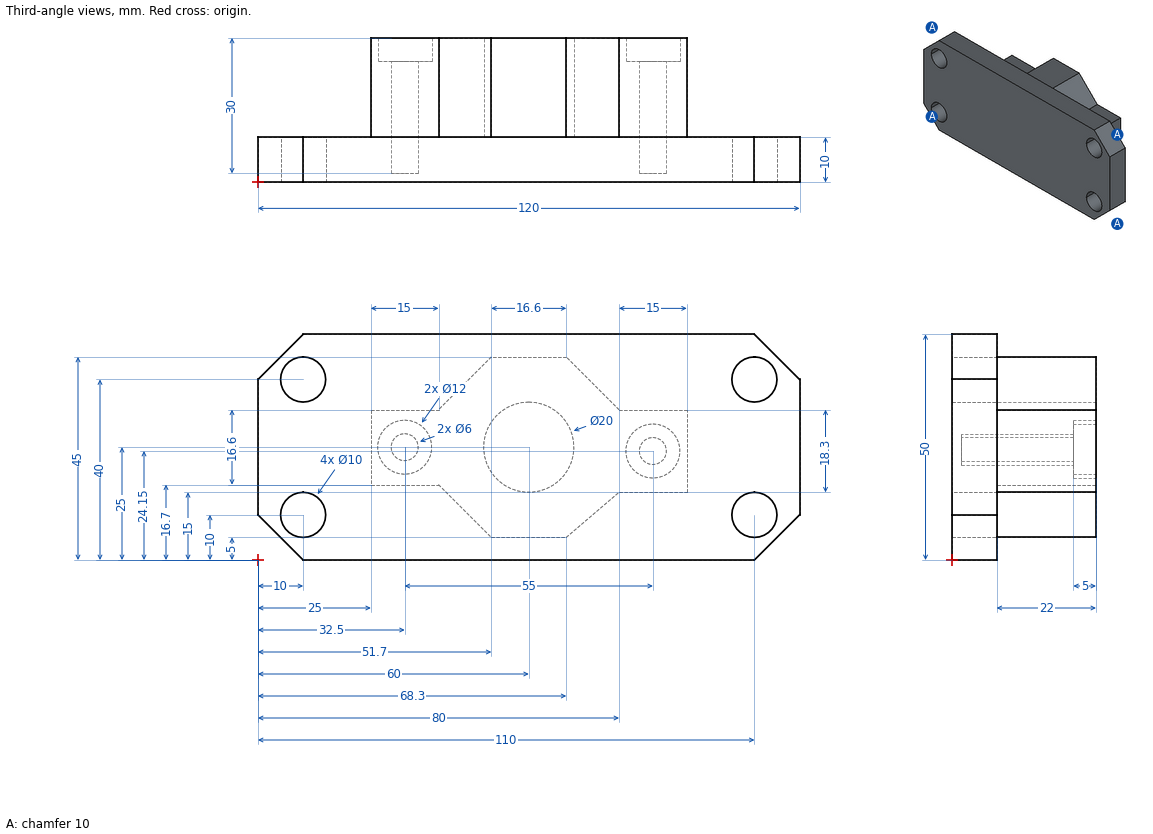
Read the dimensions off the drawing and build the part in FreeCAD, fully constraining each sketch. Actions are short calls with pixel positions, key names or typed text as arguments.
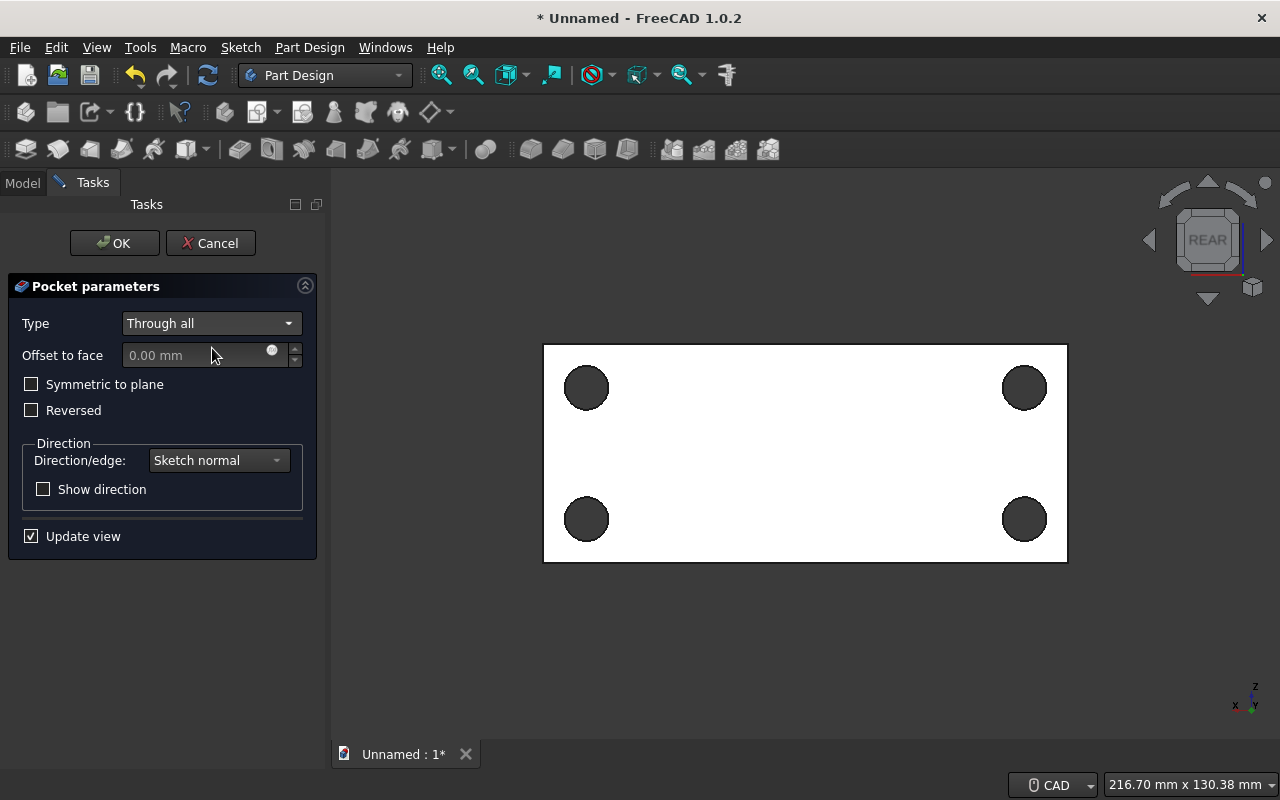
click(115, 243)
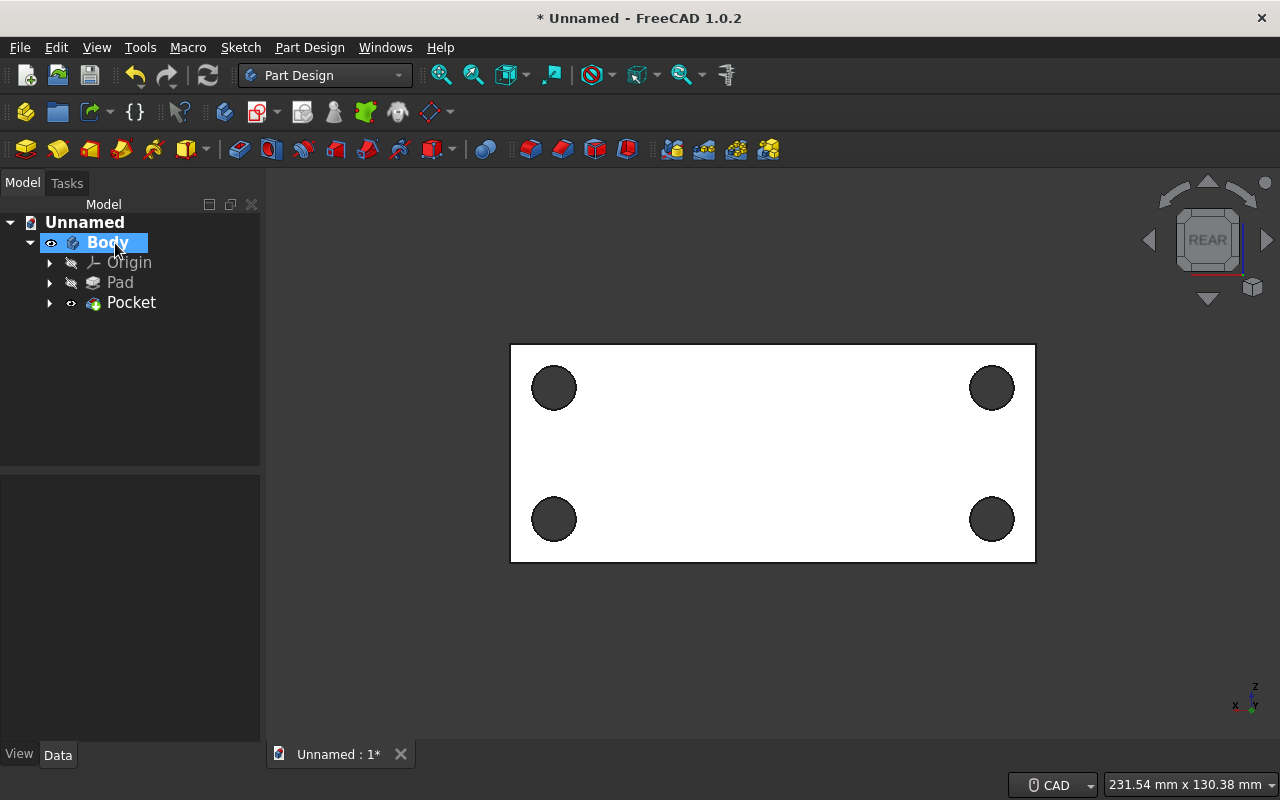
click(698, 452)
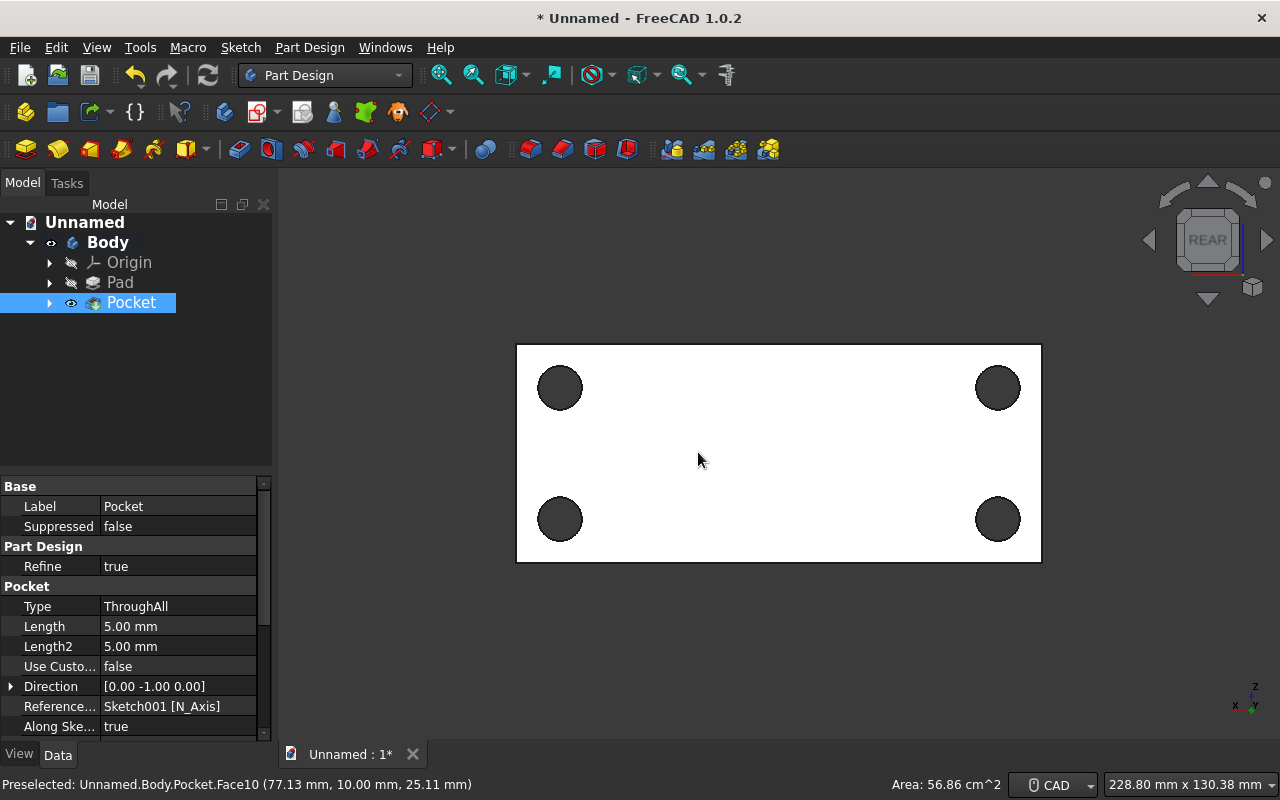
click(258, 112)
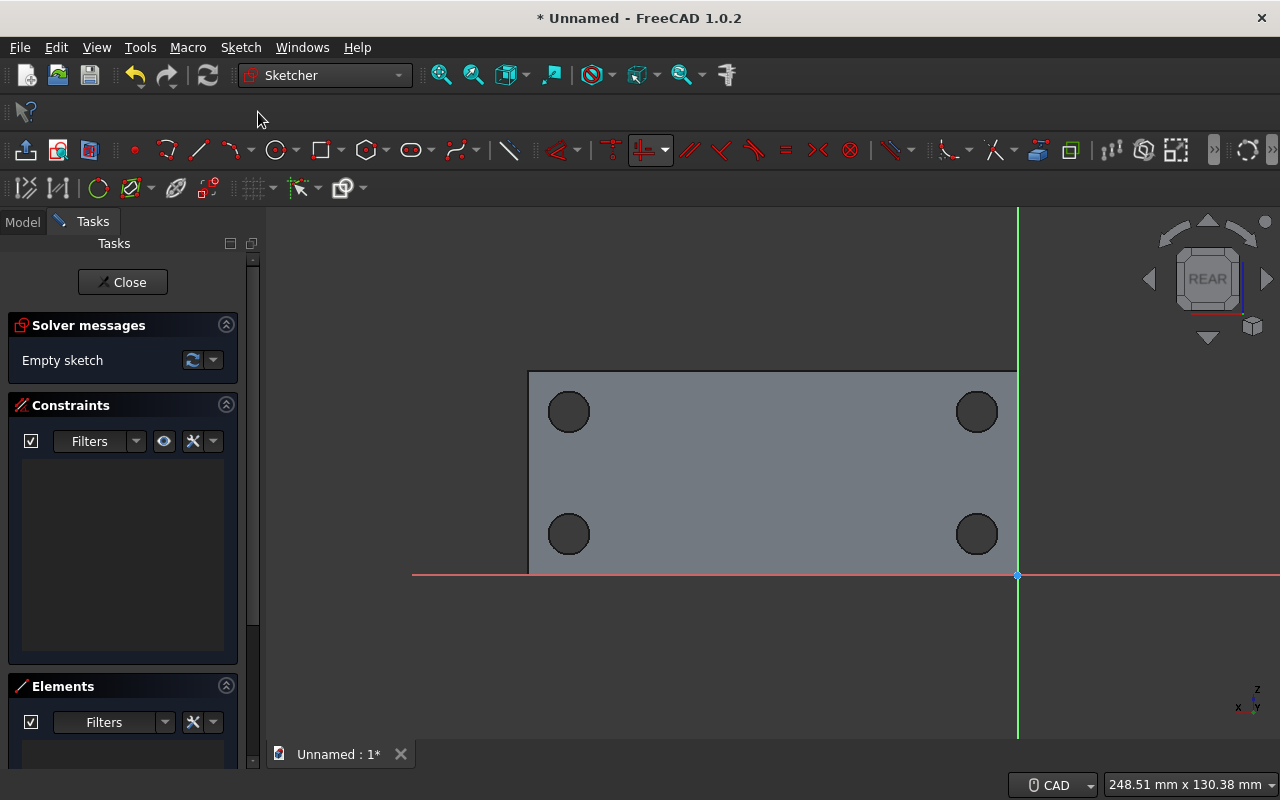
scroll(1067, 504, up, 2)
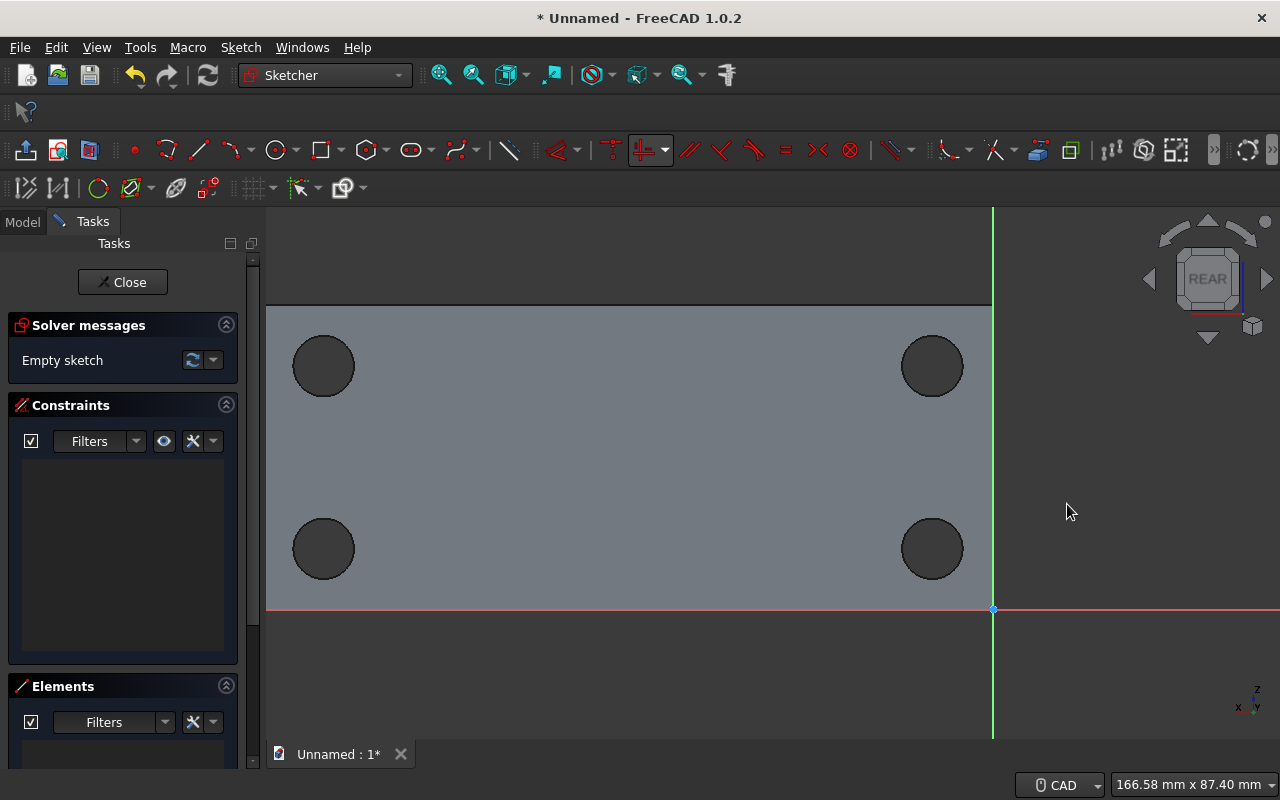
click(168, 150)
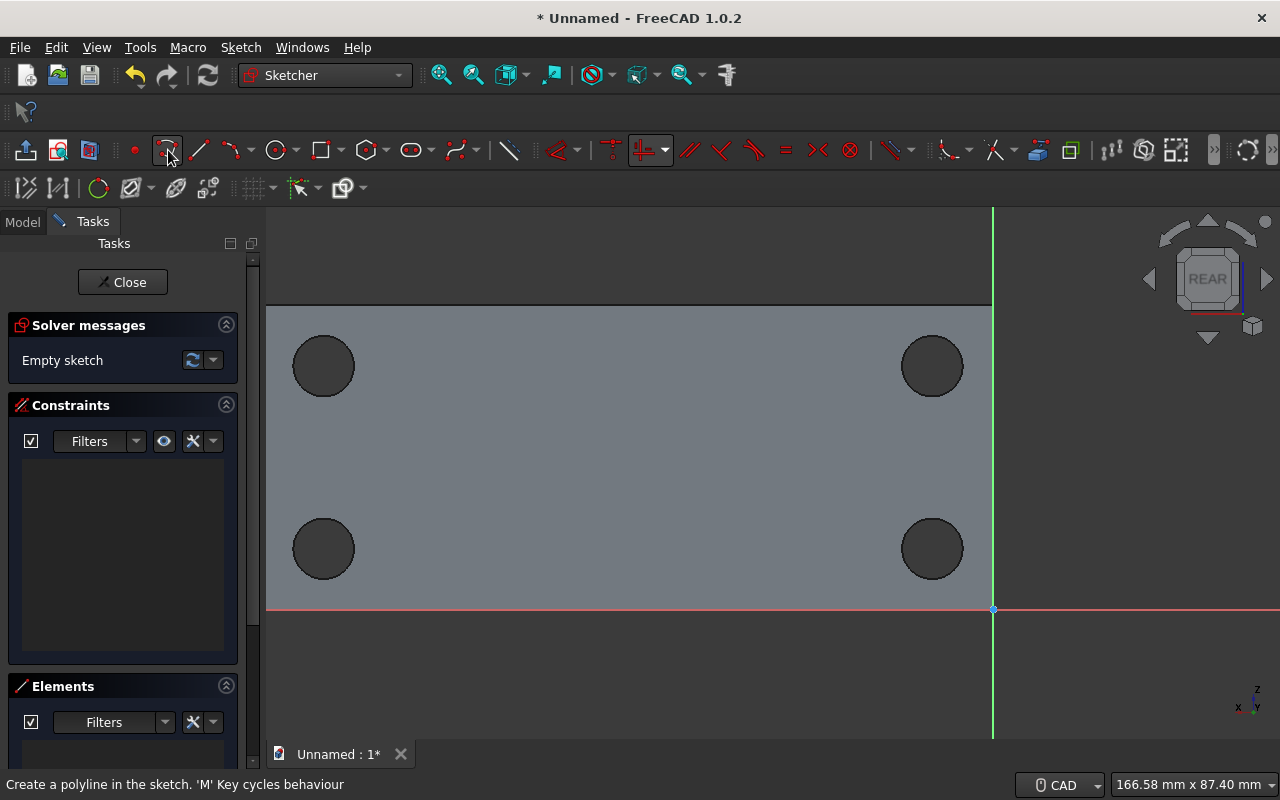
click(841, 508)
click(841, 407)
click(750, 407)
click(679, 336)
click(577, 336)
click(506, 407)
click(415, 407)
click(415, 518)
click(506, 518)
click(577, 579)
click(679, 579)
click(750, 508)
click(841, 509)
key(Escape)
key(Escape)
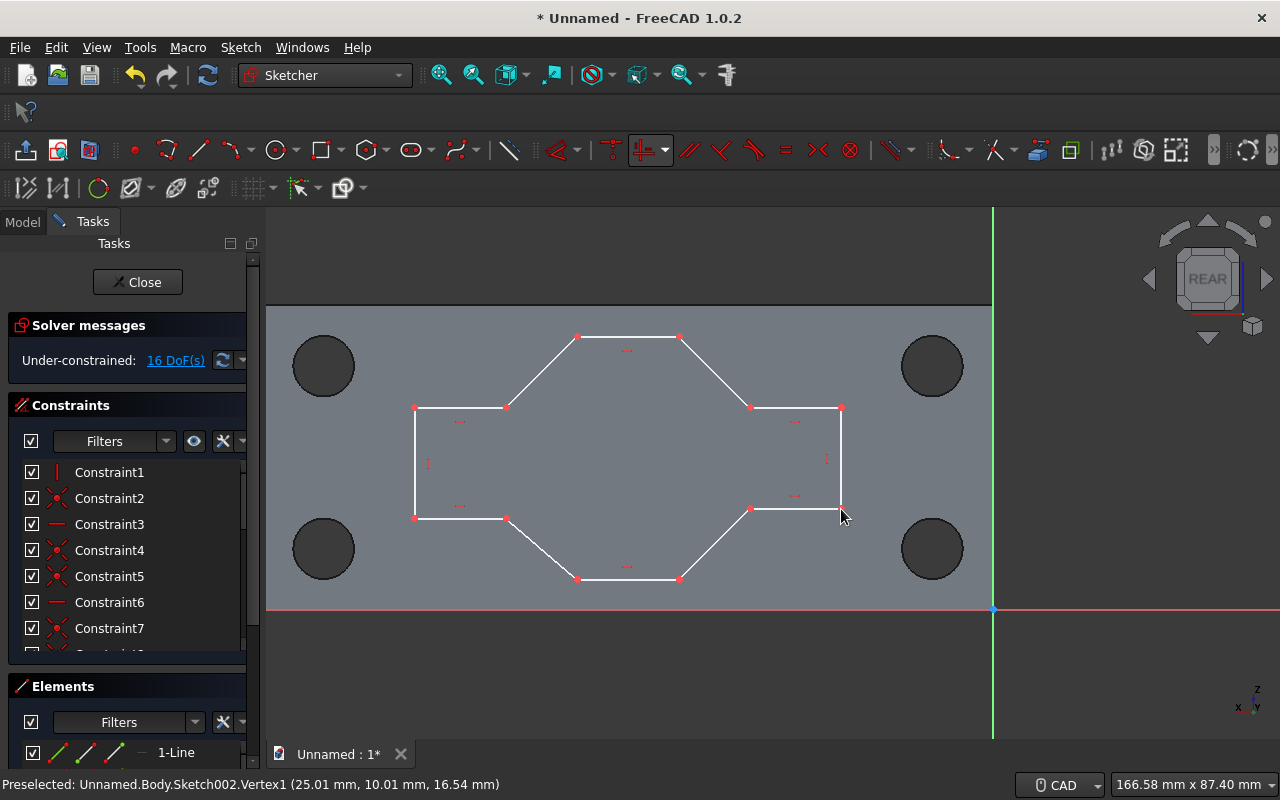
click(556, 150)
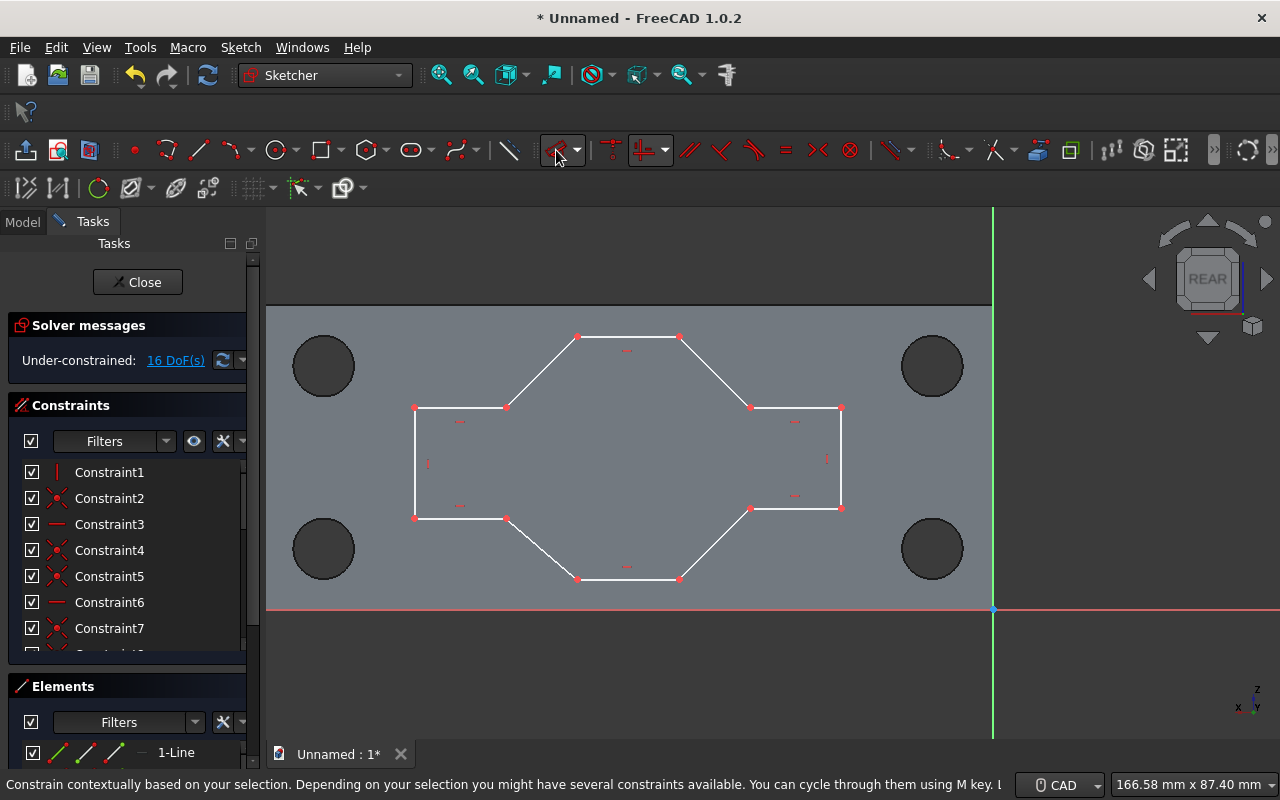
click(814, 408)
click(796, 374)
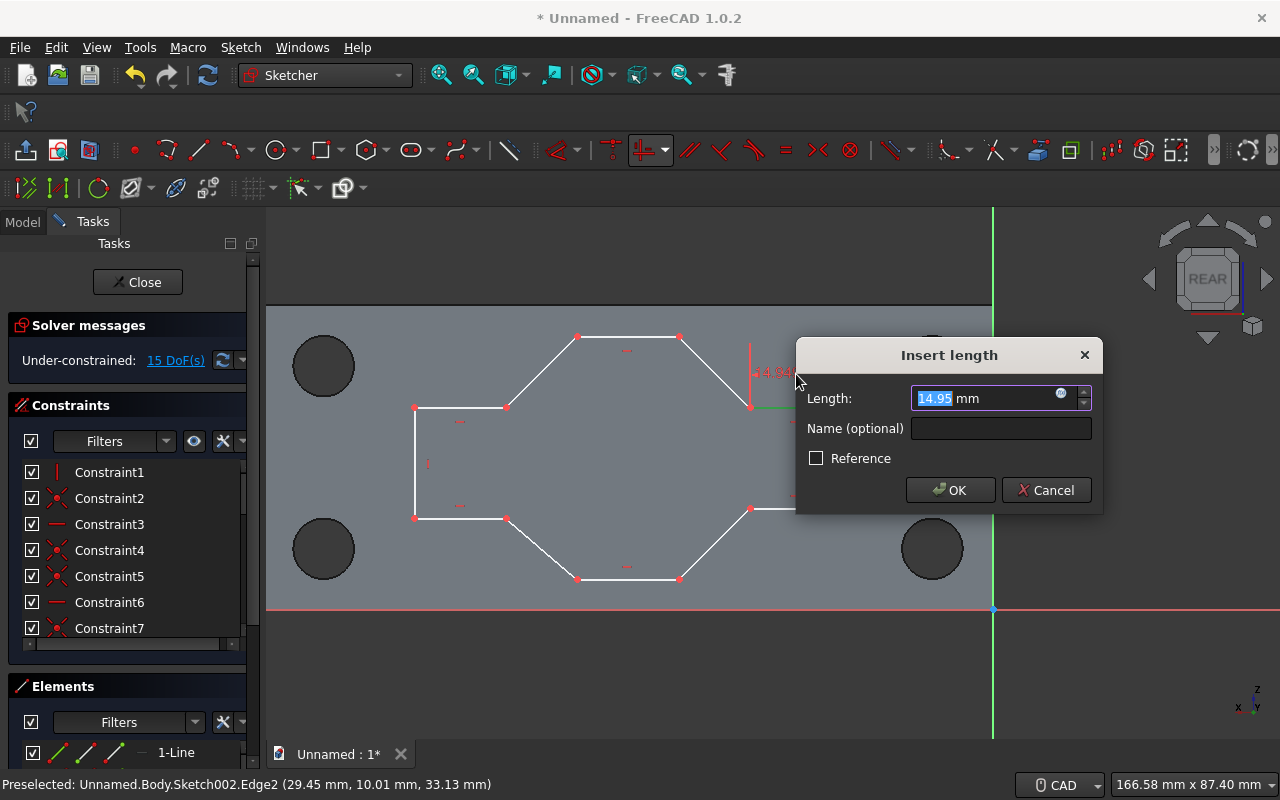
text(15)
key(Return)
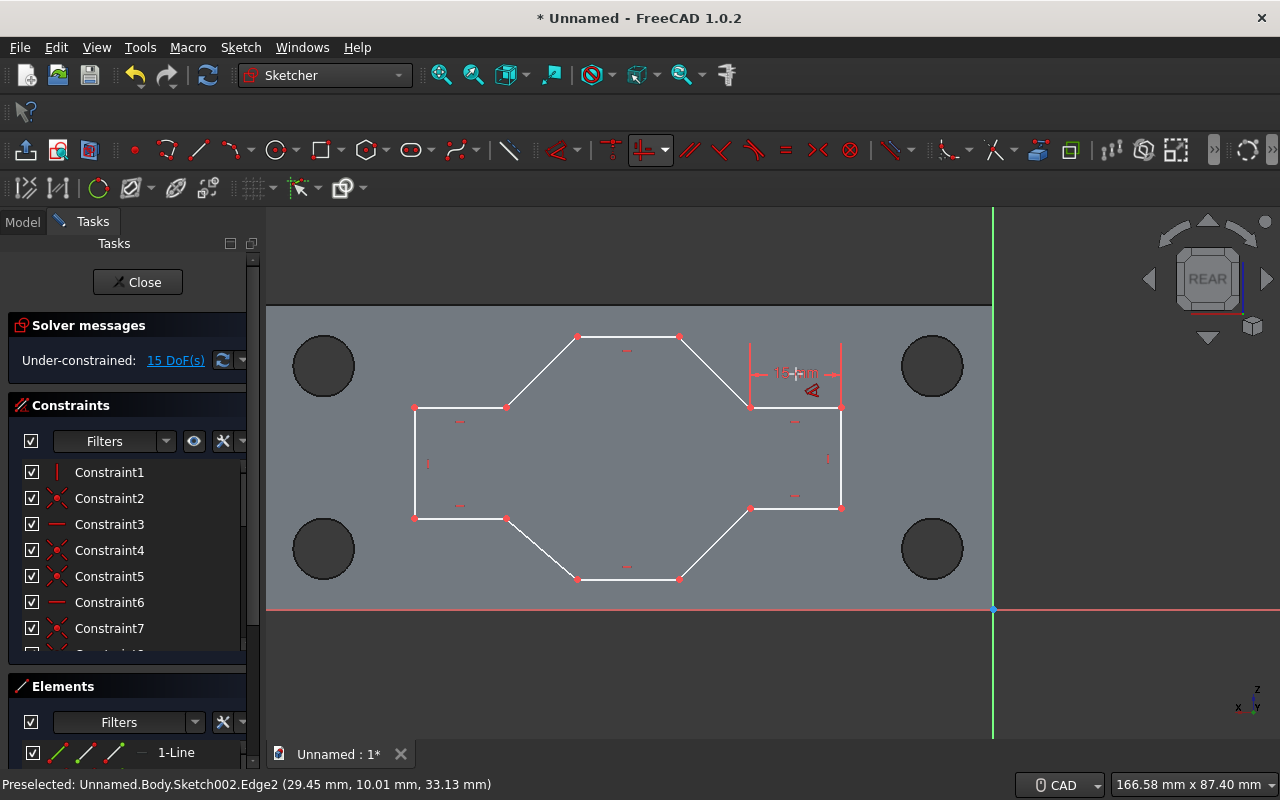
click(479, 408)
click(461, 374)